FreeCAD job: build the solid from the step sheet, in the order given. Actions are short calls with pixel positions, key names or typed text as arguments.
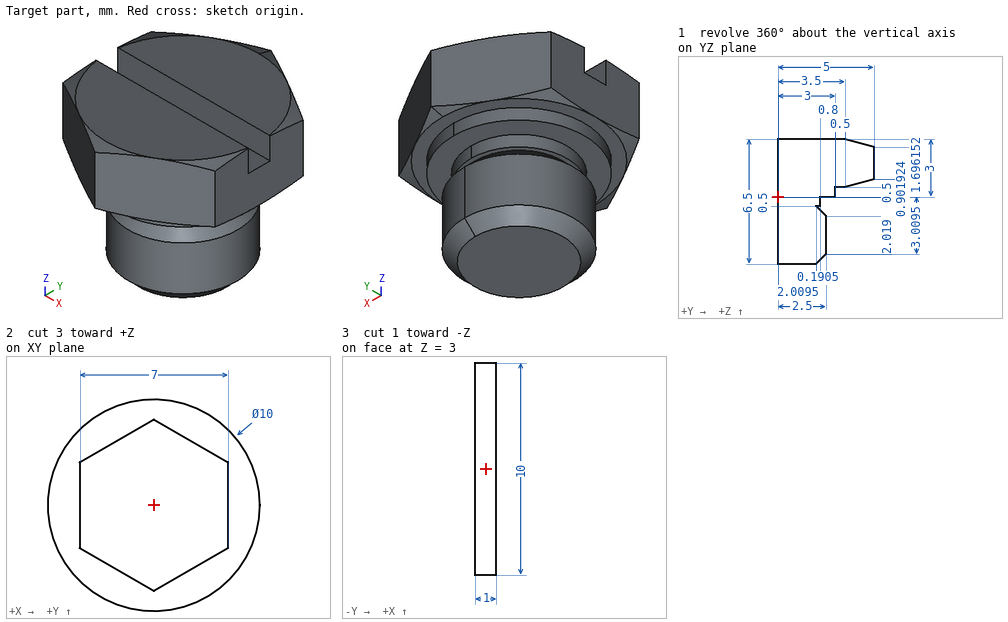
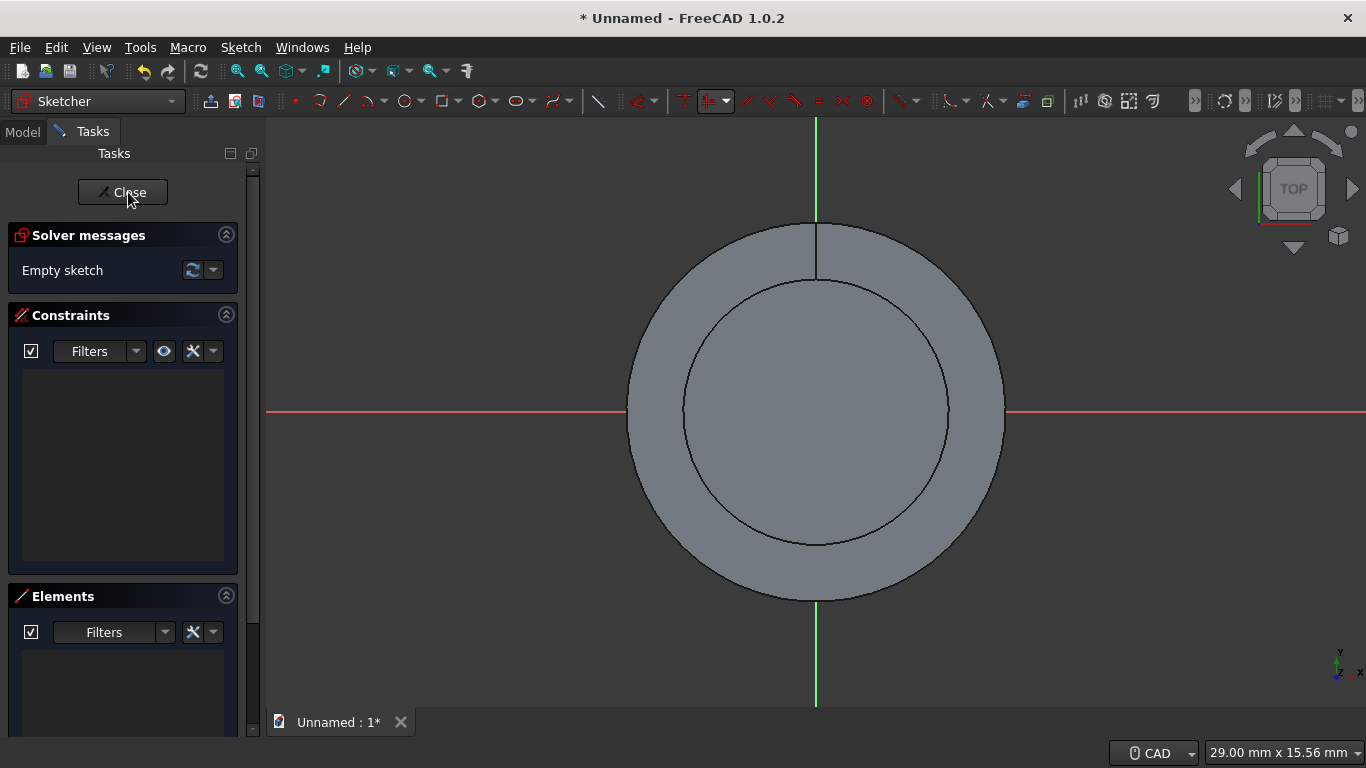
click(260, 102)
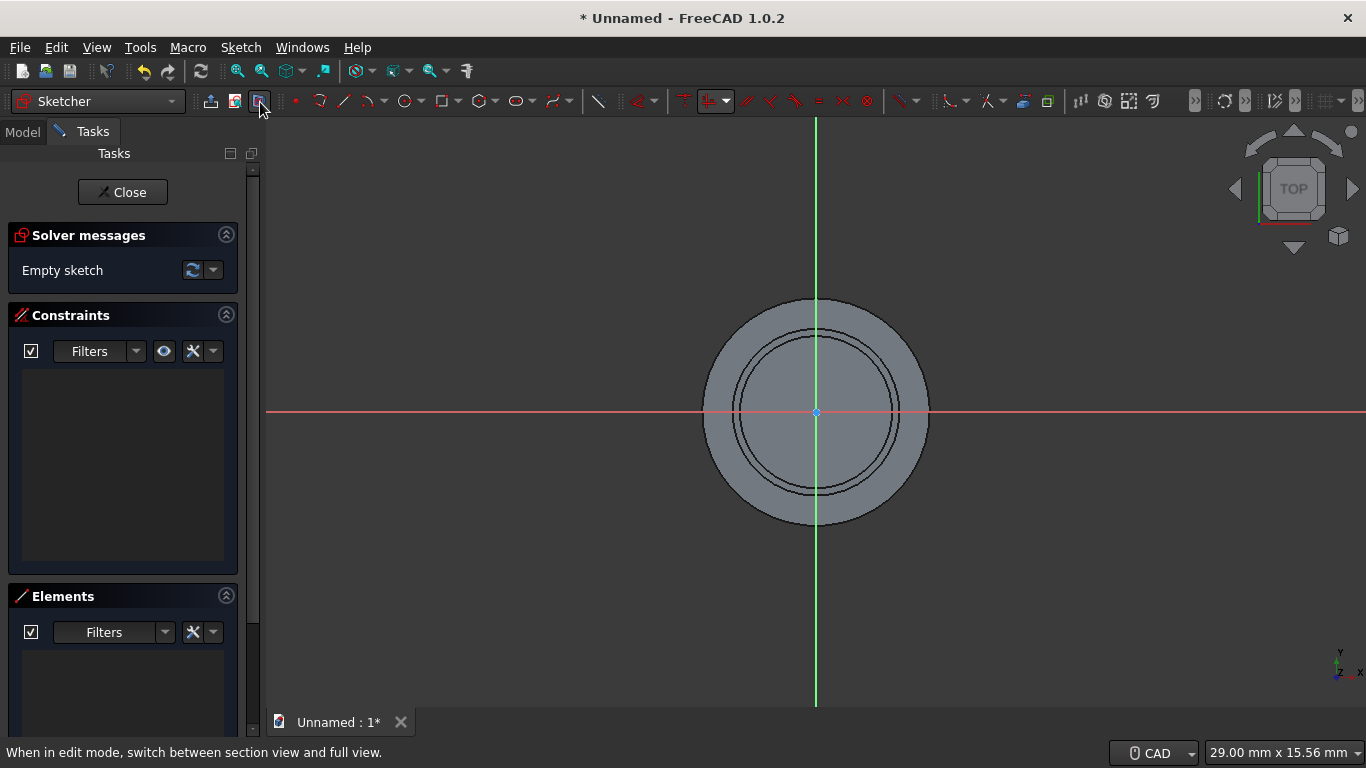
click(480, 102)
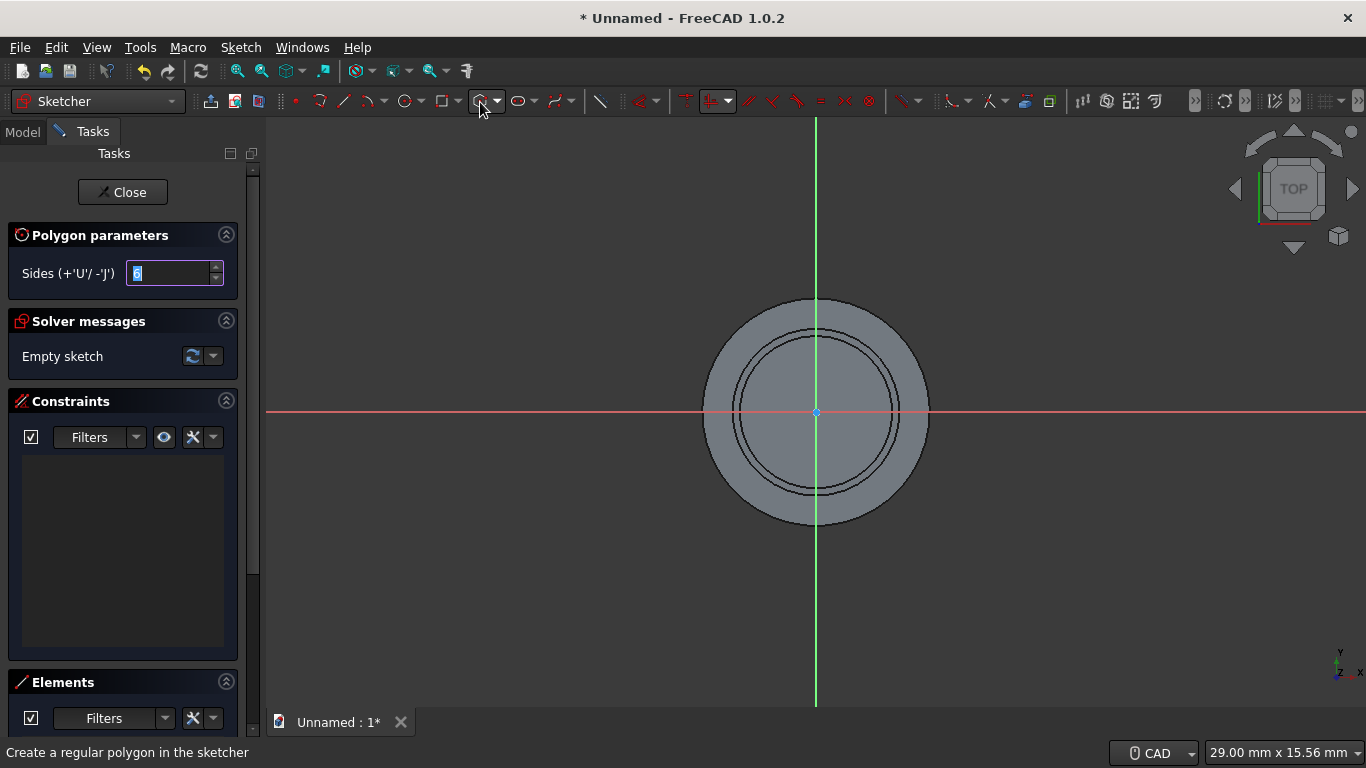
click(816, 412)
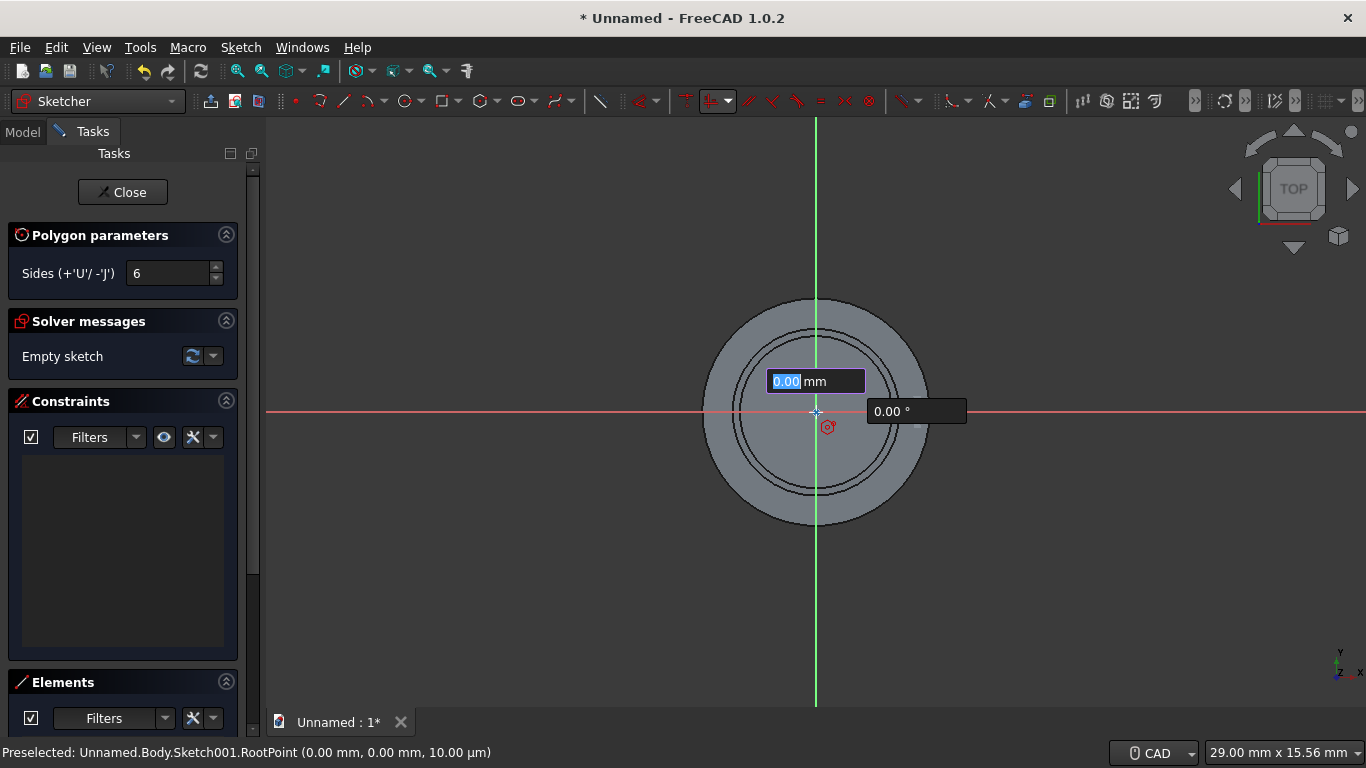
click(816, 259)
key(Escape)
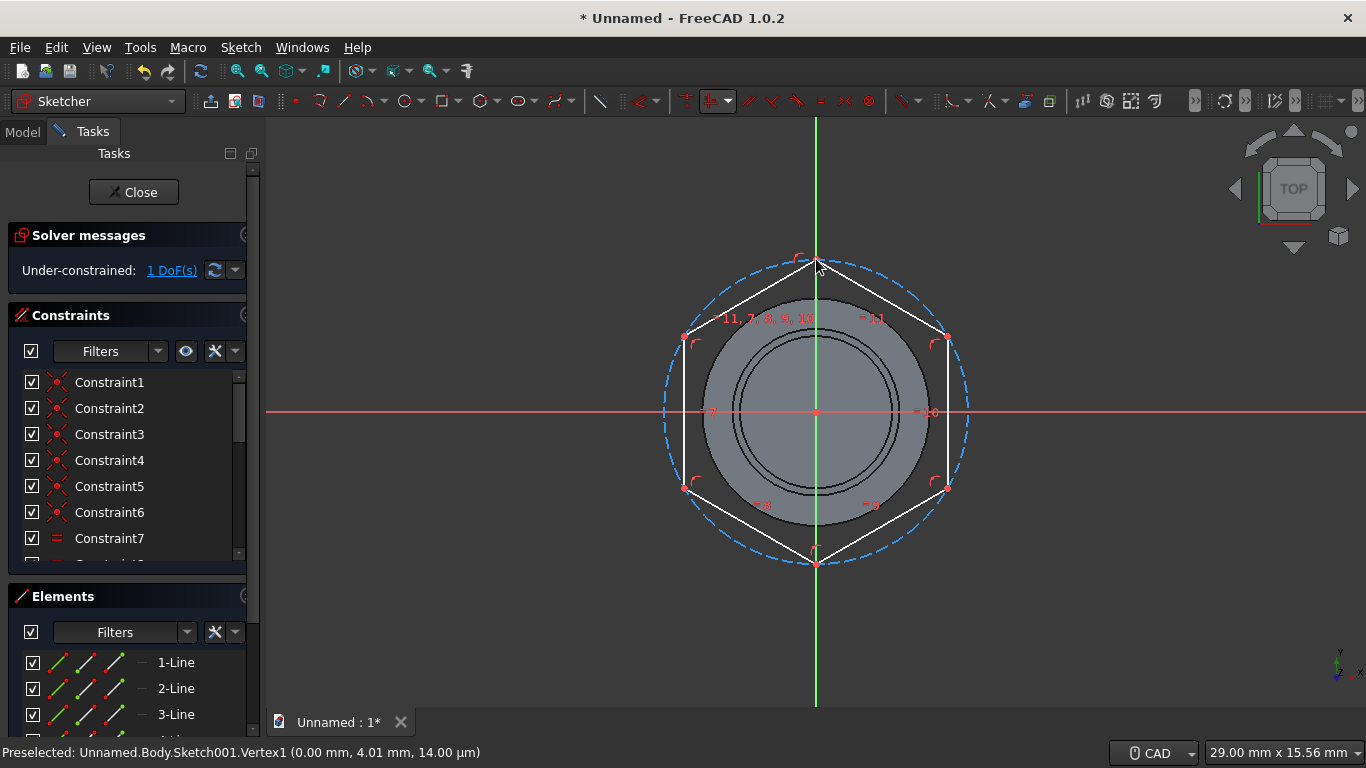
click(406, 102)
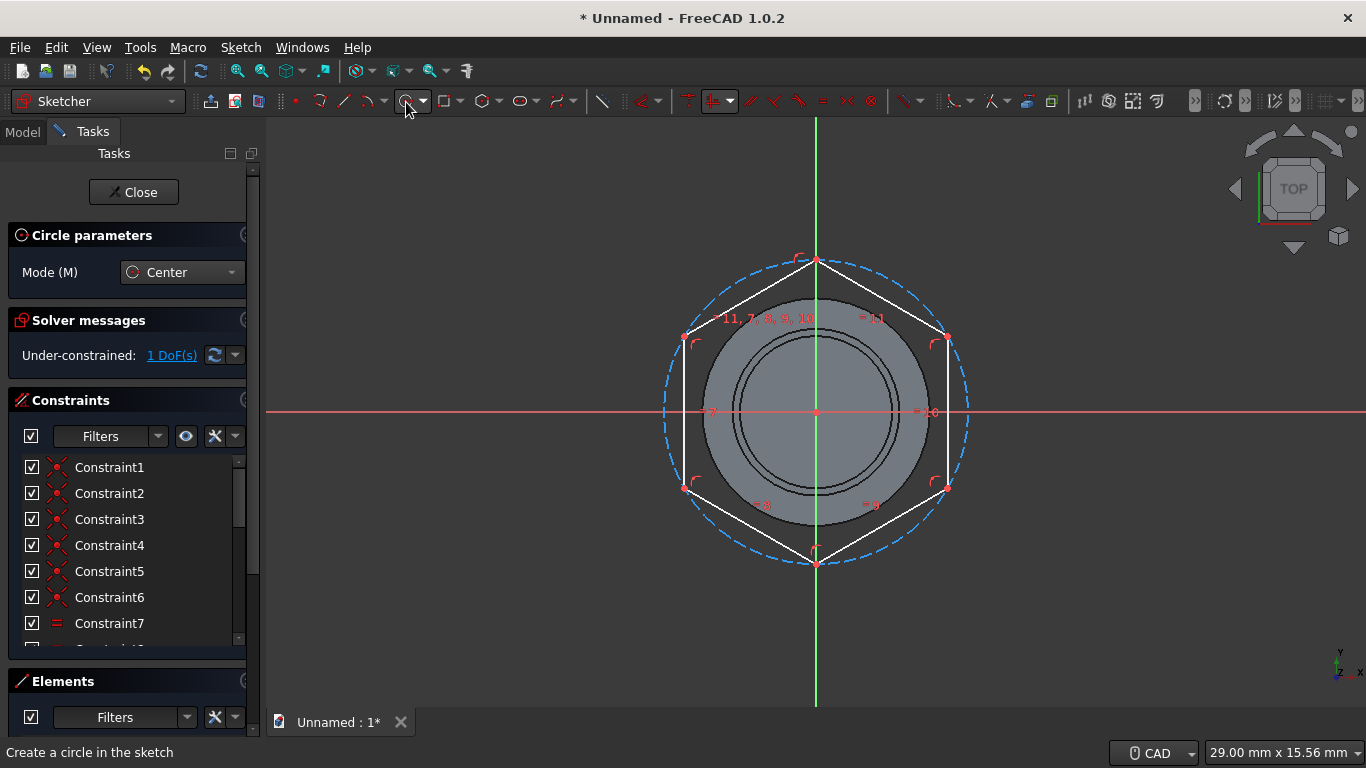
click(816, 412)
click(950, 278)
key(Escape)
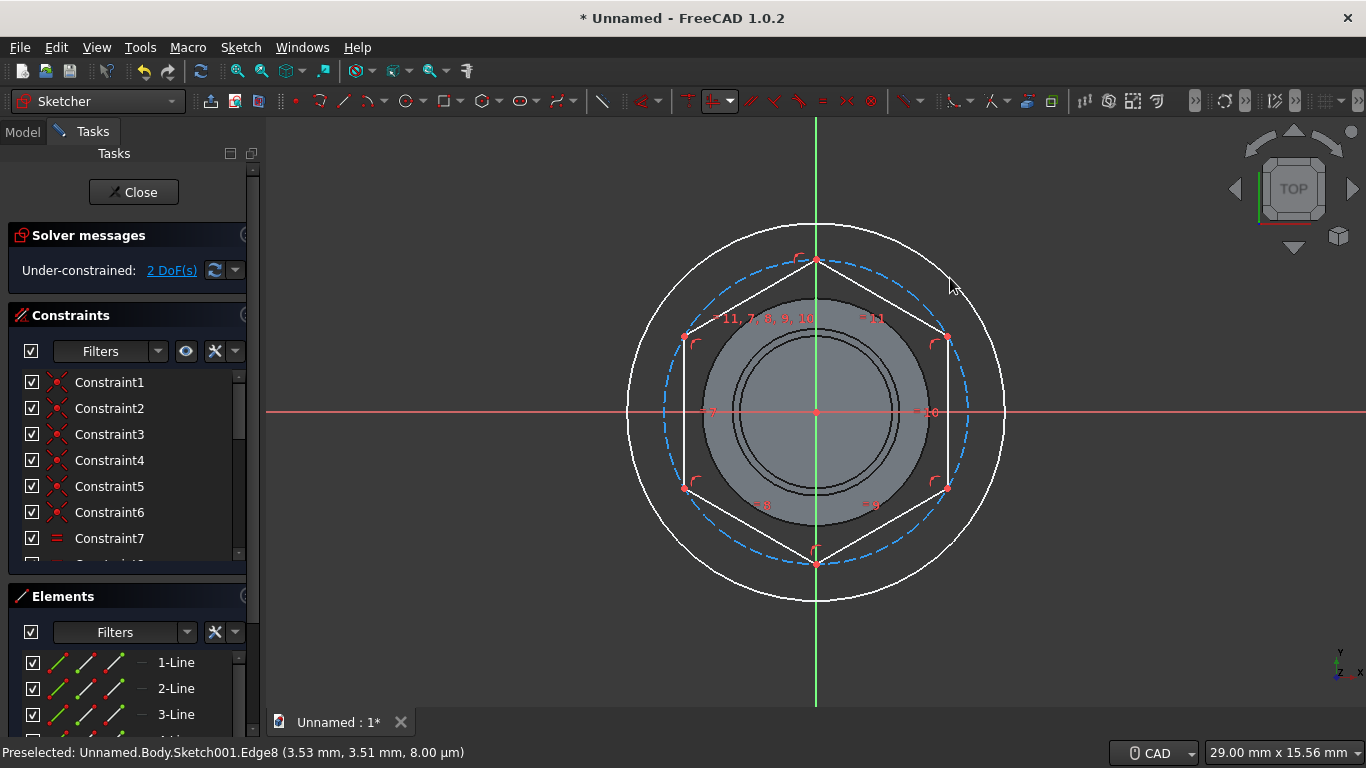
key(d)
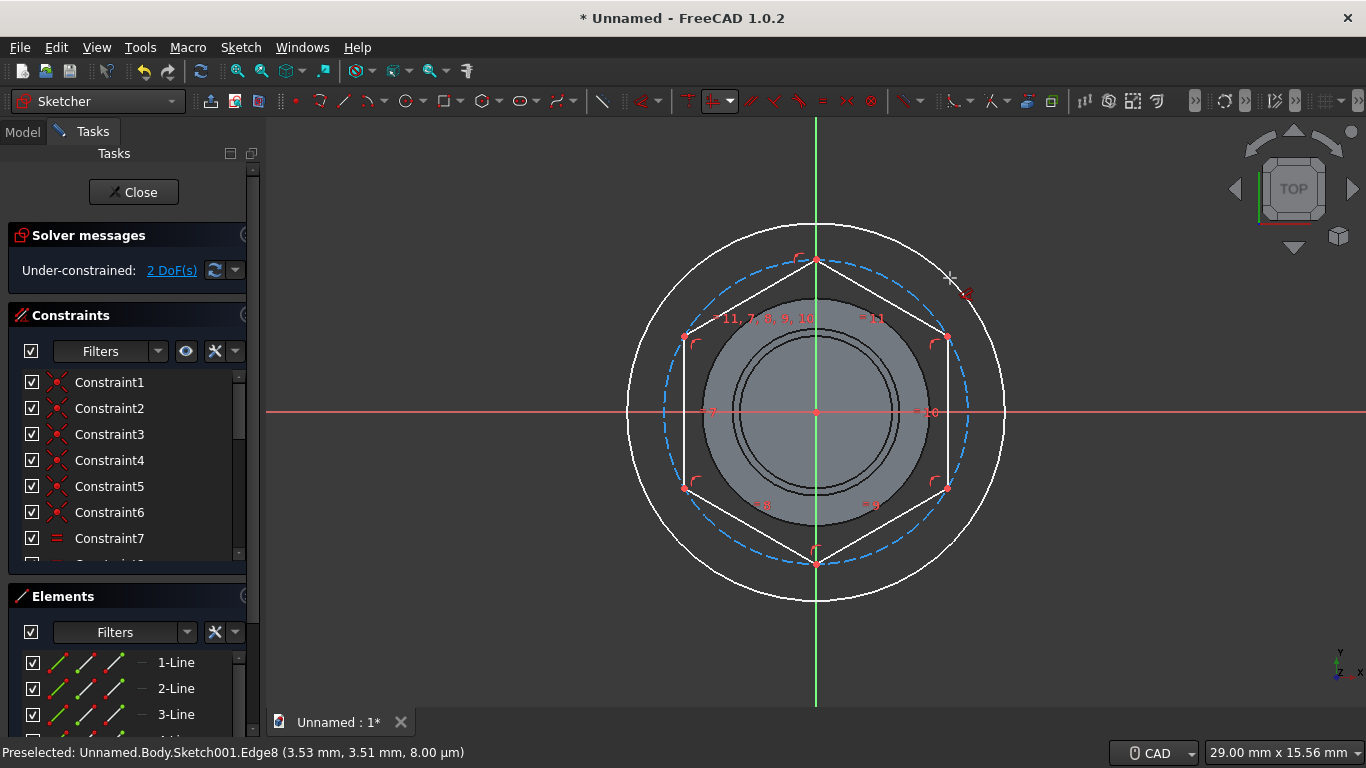
click(949, 278)
click(972, 255)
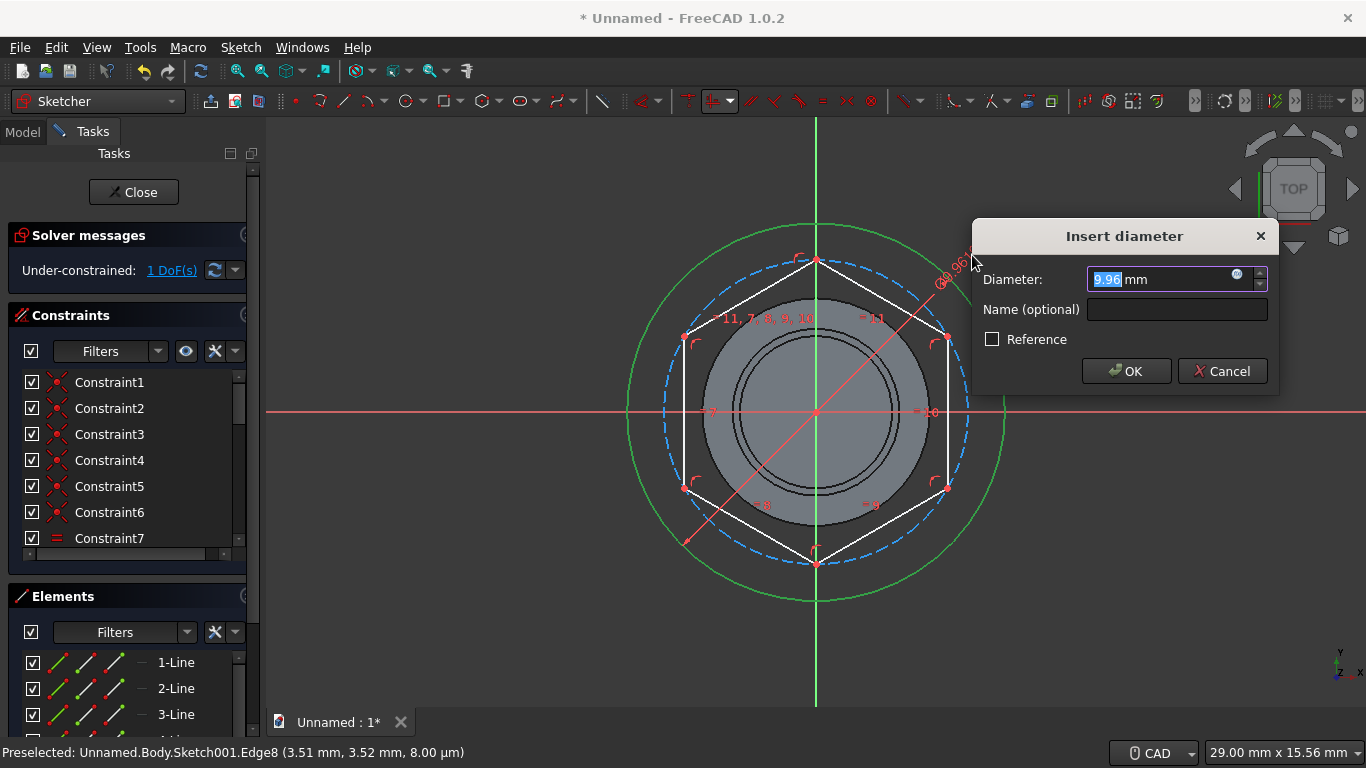
text(10)
key(Return)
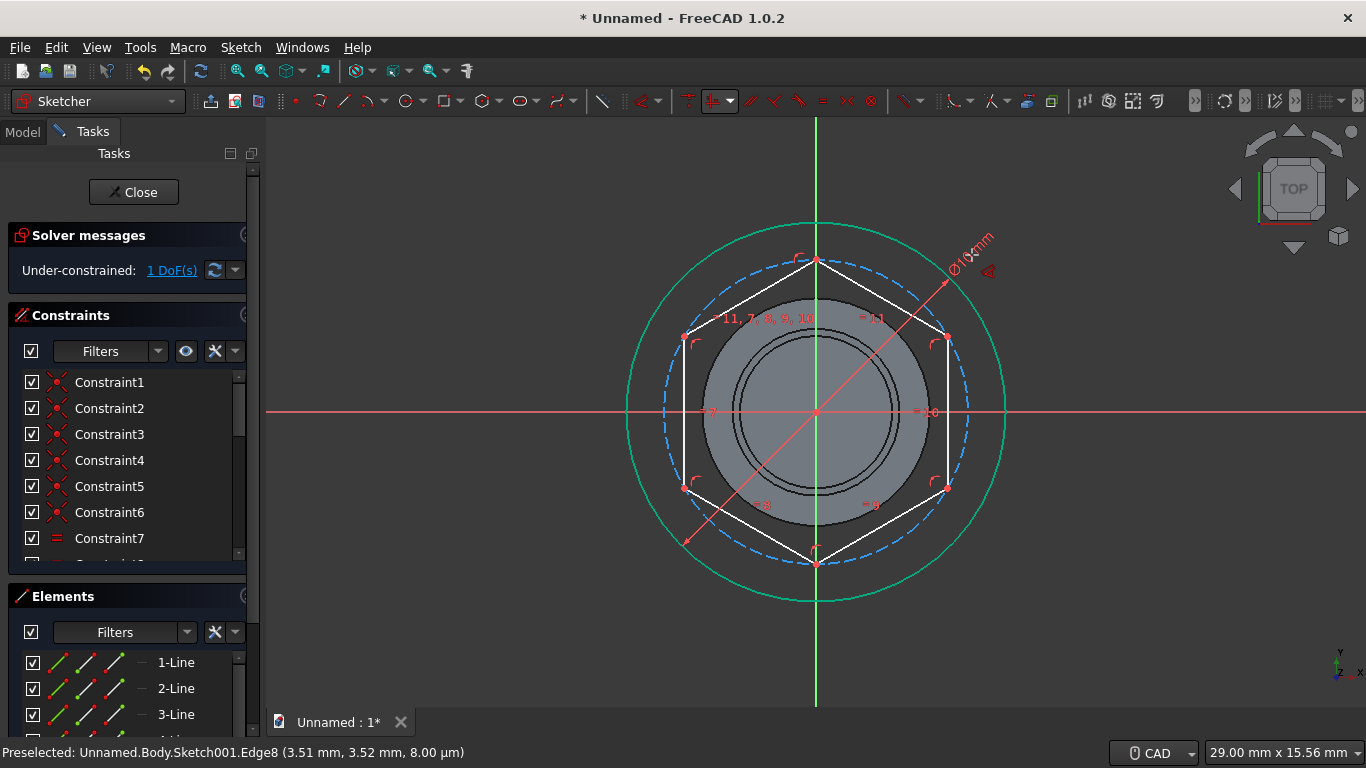
click(684, 336)